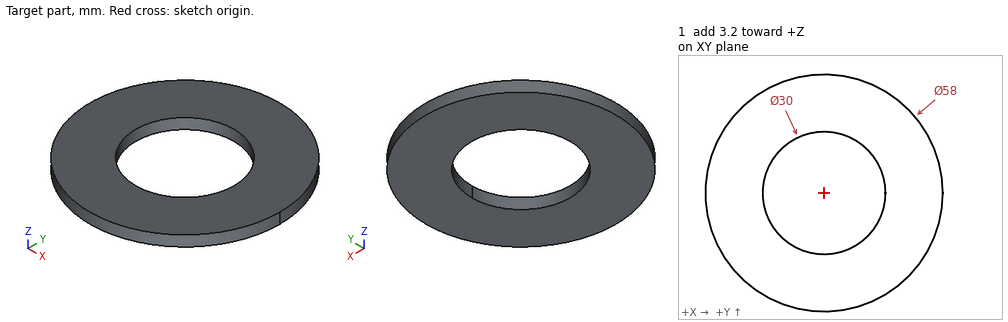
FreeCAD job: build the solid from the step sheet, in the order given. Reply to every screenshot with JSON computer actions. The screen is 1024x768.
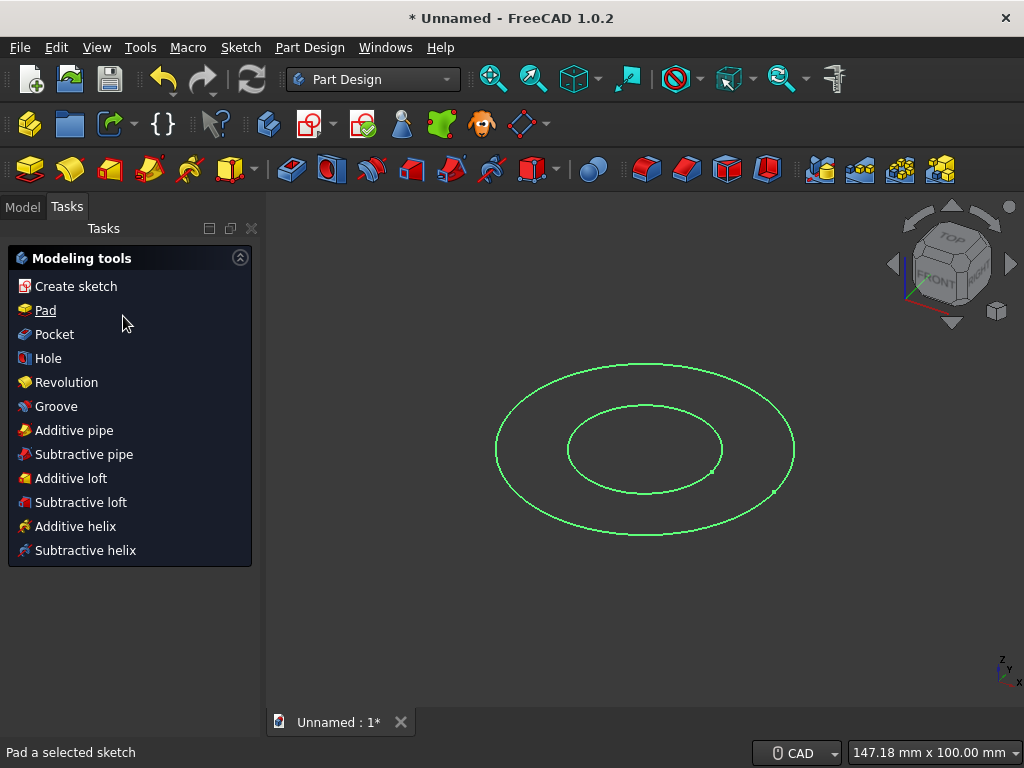
{"action": "left_click", "coordinate": [30, 170]}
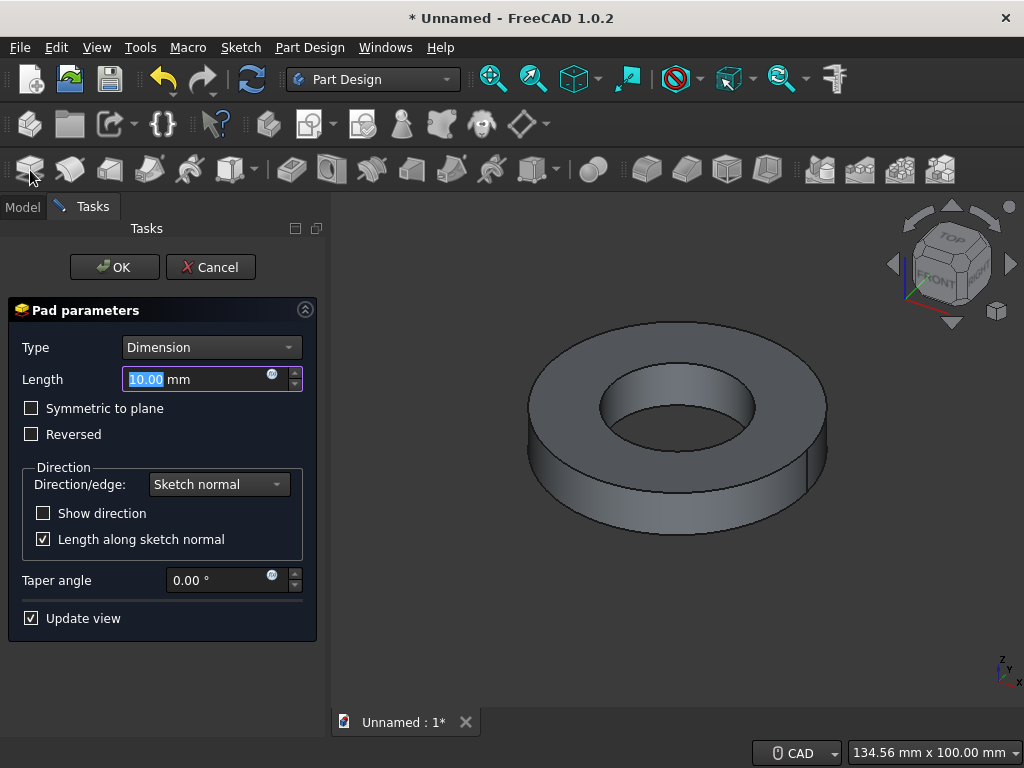
{"action": "type", "text": "3.2"}
{"action": "key", "text": "Tab"}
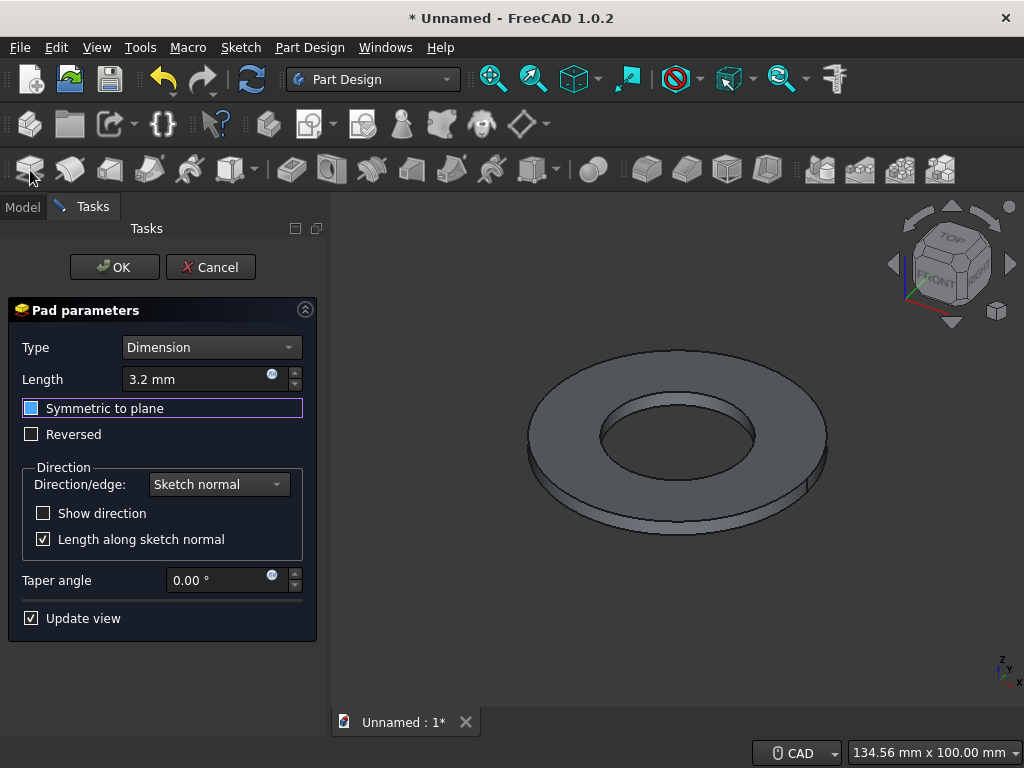
{"action": "left_click", "coordinate": [115, 267]}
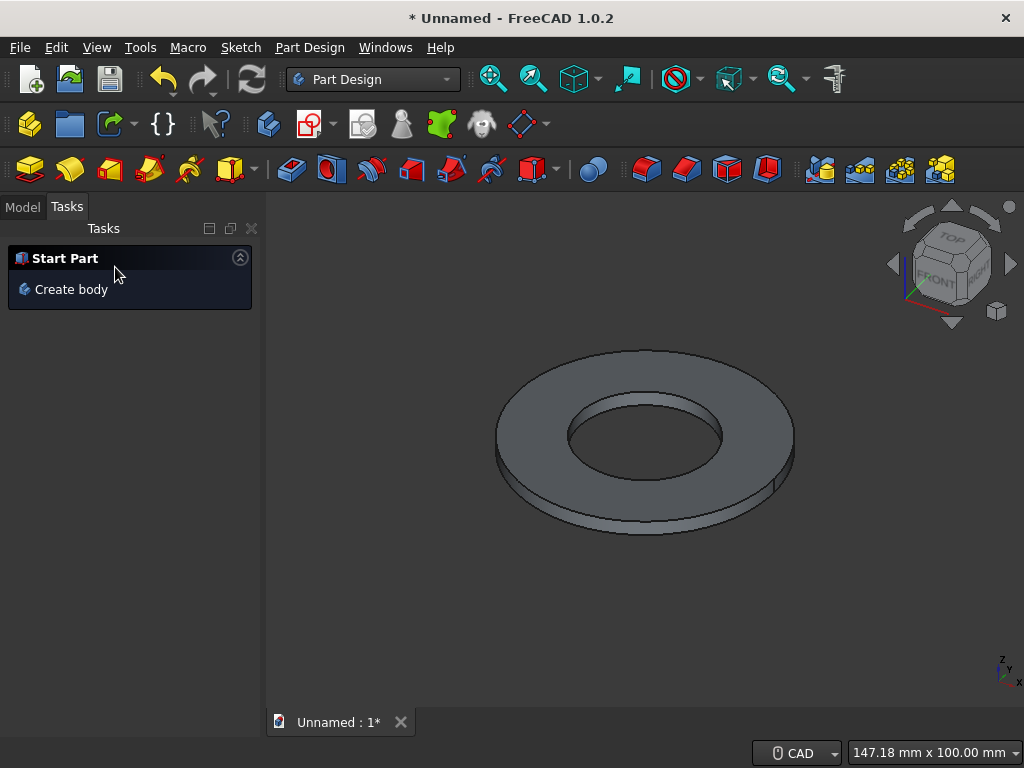
{"action": "key", "text": "0"}